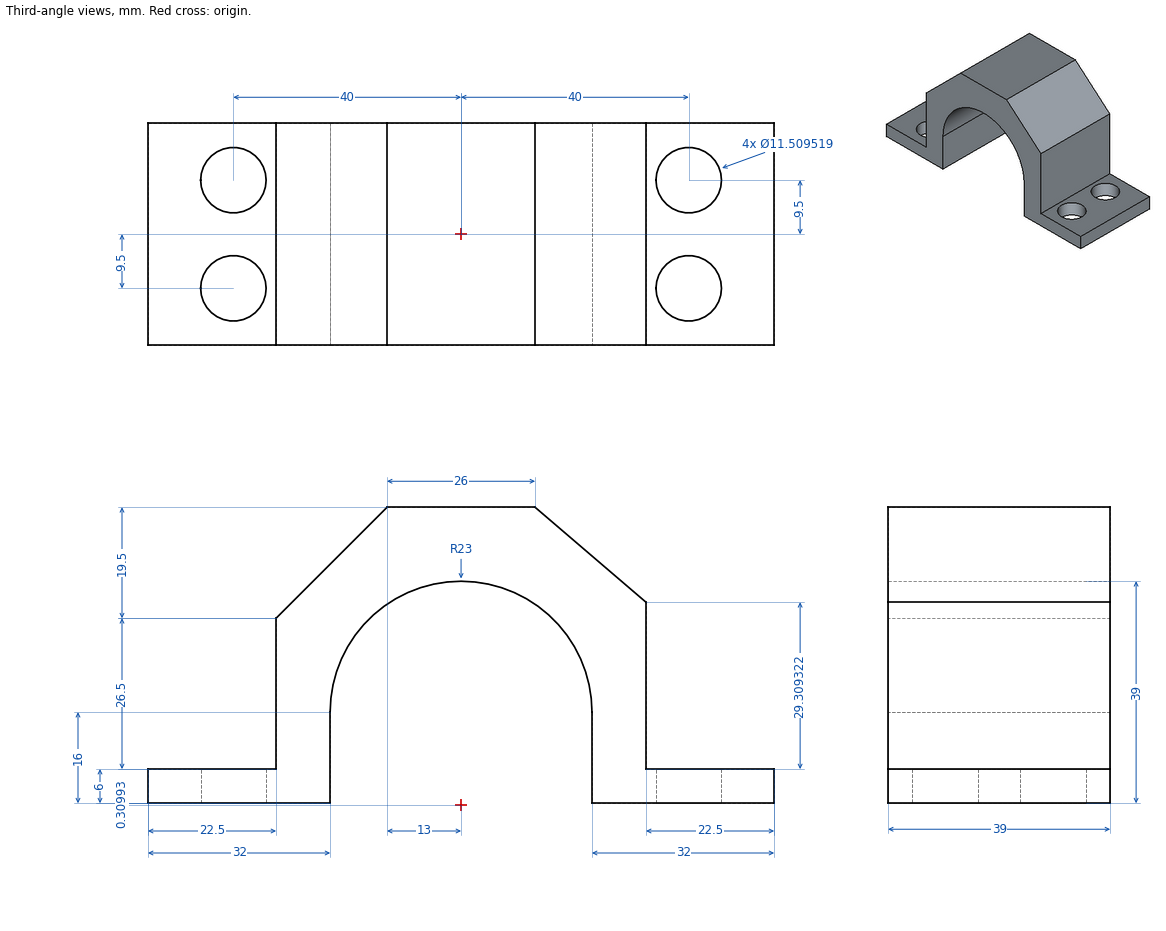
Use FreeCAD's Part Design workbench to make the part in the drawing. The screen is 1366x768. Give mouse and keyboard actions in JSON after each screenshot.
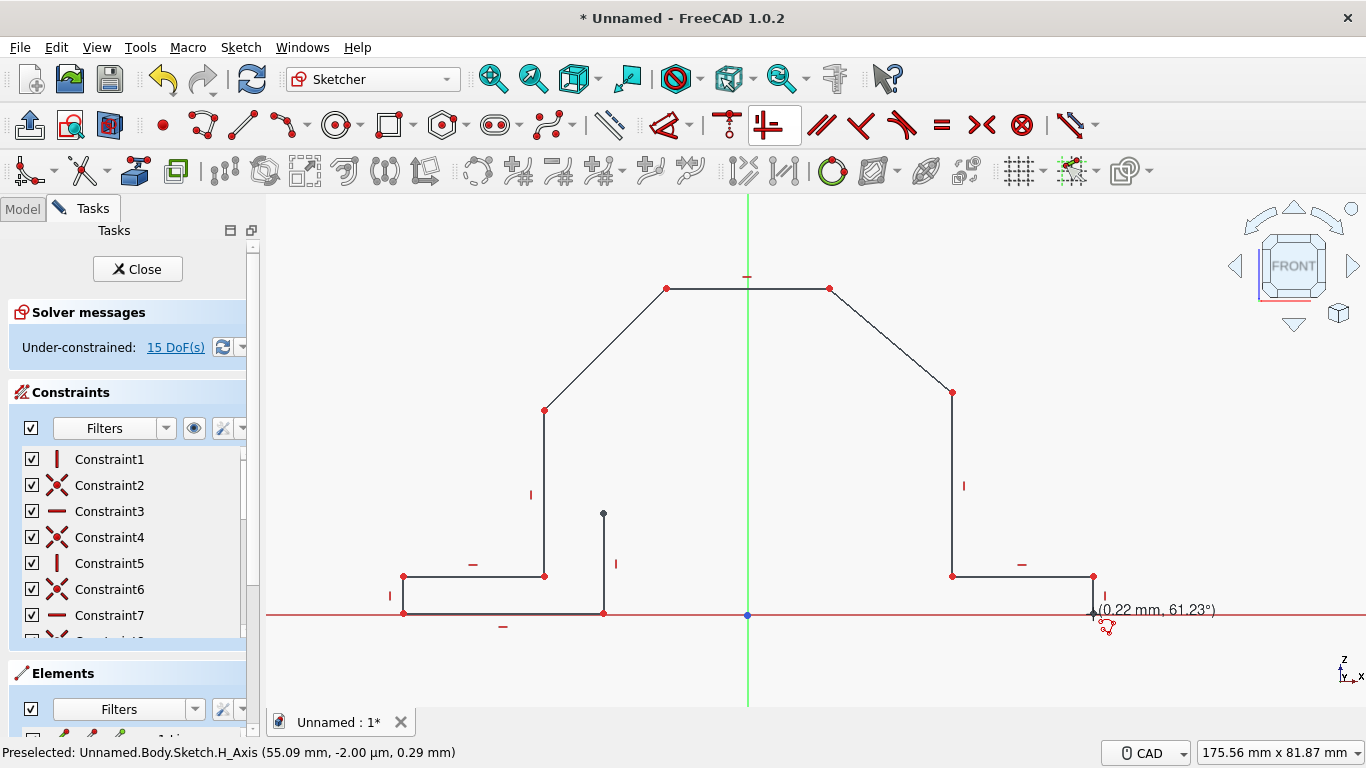
{"action": "scroll", "coordinate": [892, 614], "scroll_direction": "up", "scroll_amount": 11}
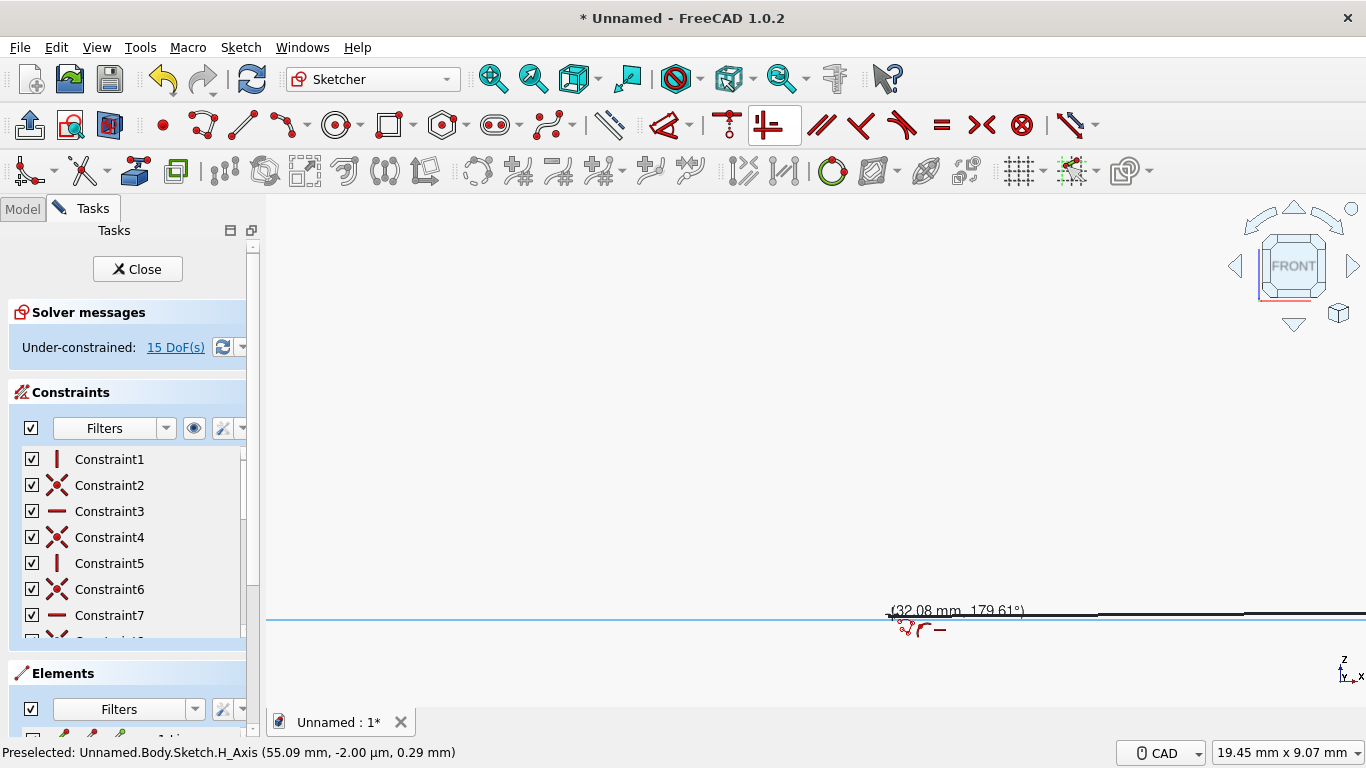
{"action": "left_click", "coordinate": [888, 603]}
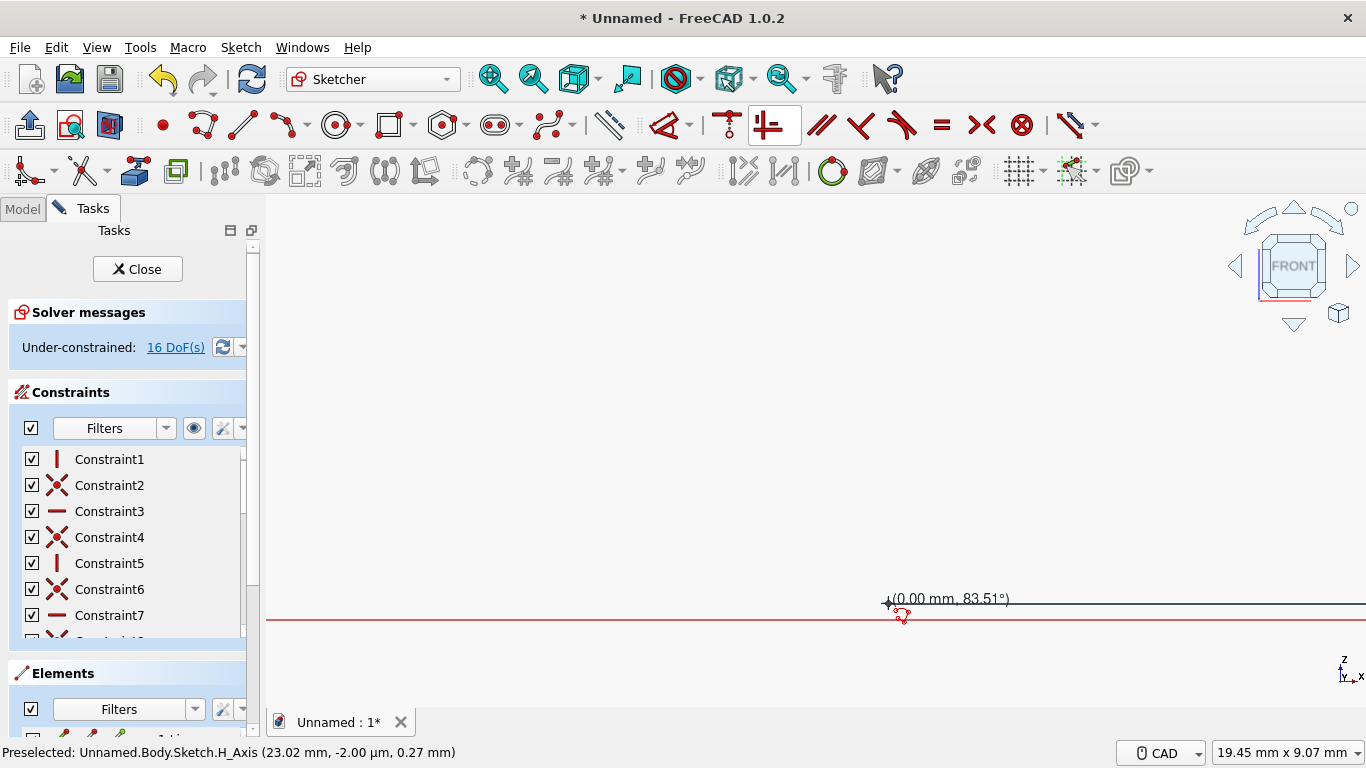
{"action": "scroll", "coordinate": [892, 614], "scroll_direction": "down", "scroll_amount": 11}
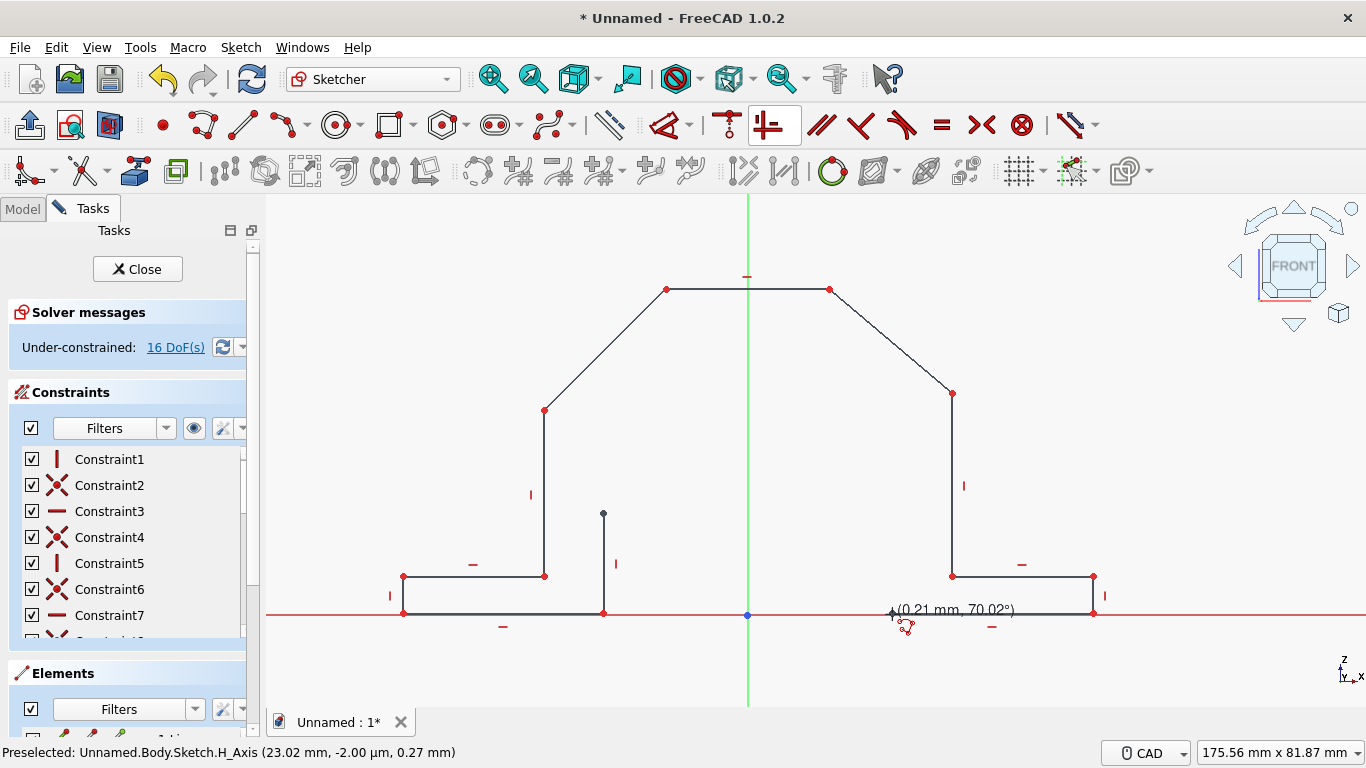
{"action": "left_click", "coordinate": [892, 513]}
{"action": "right_click", "coordinate": [892, 513]}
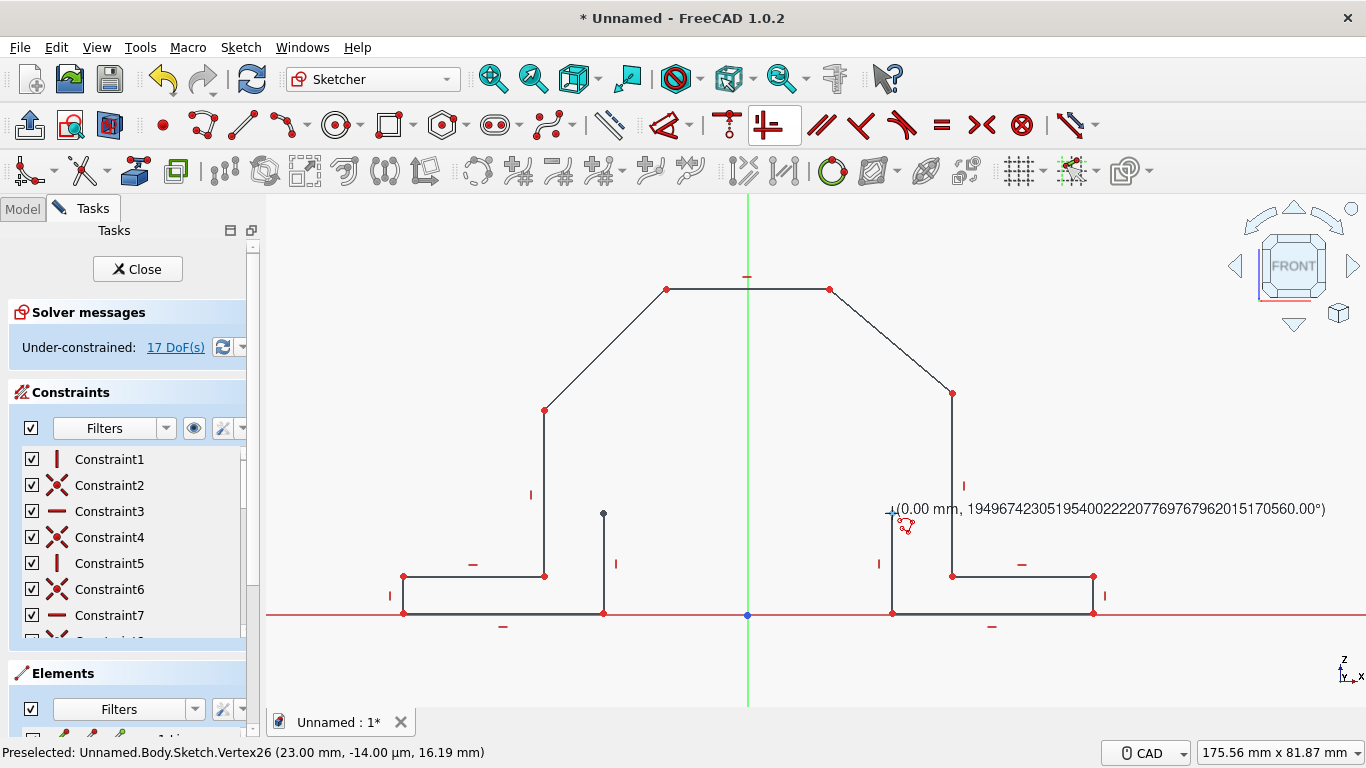
{"action": "left_click", "coordinate": [284, 126]}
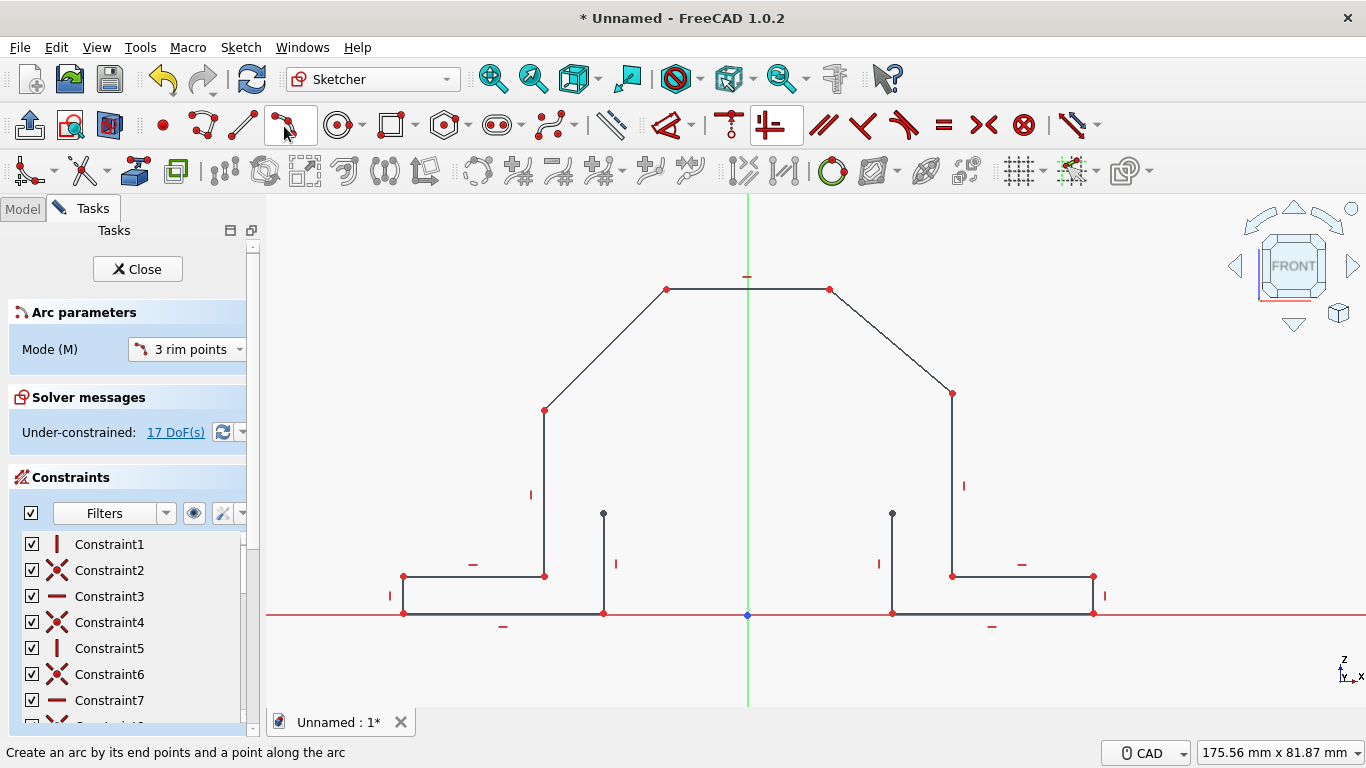
{"action": "left_click", "coordinate": [892, 514]}
{"action": "left_click", "coordinate": [604, 514]}
{"action": "left_click", "coordinate": [792, 376]}
{"action": "key", "text": "Escape"}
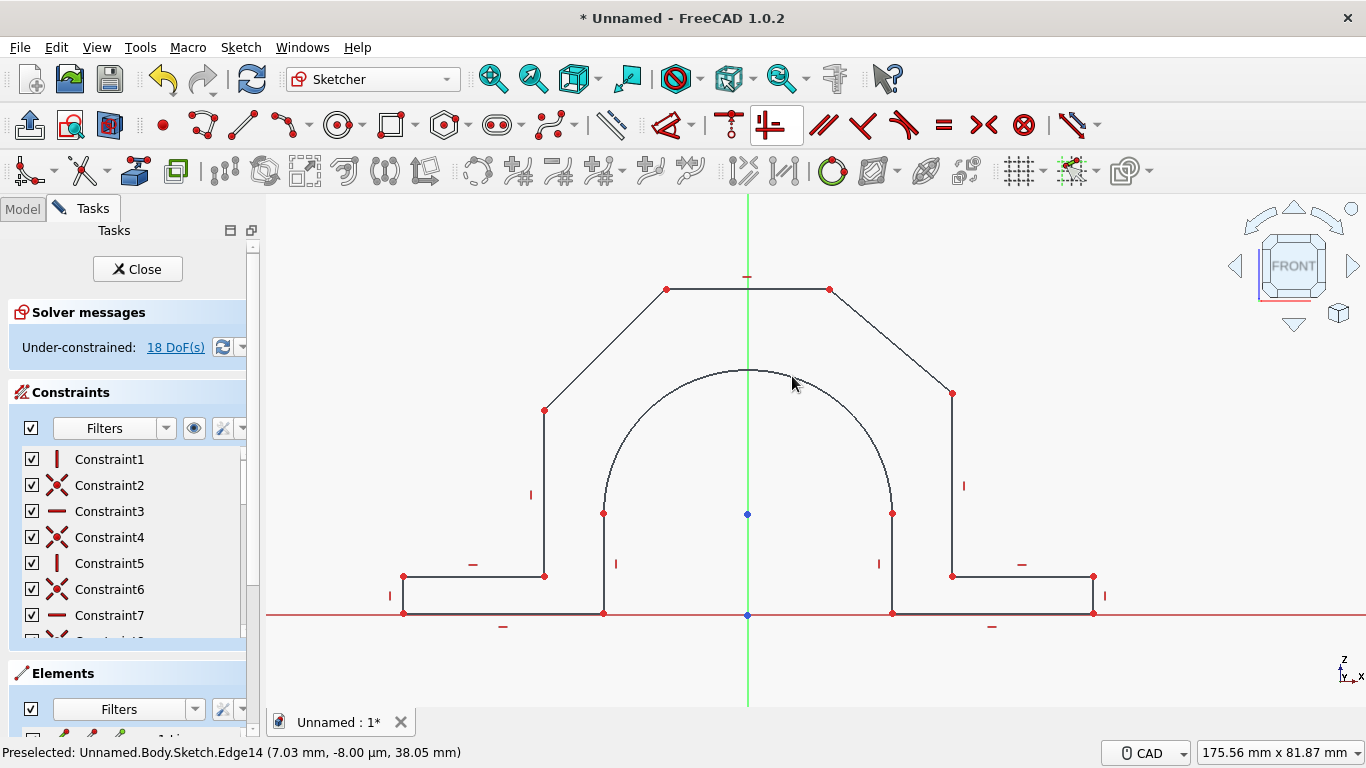
{"action": "left_click", "coordinate": [604, 544]}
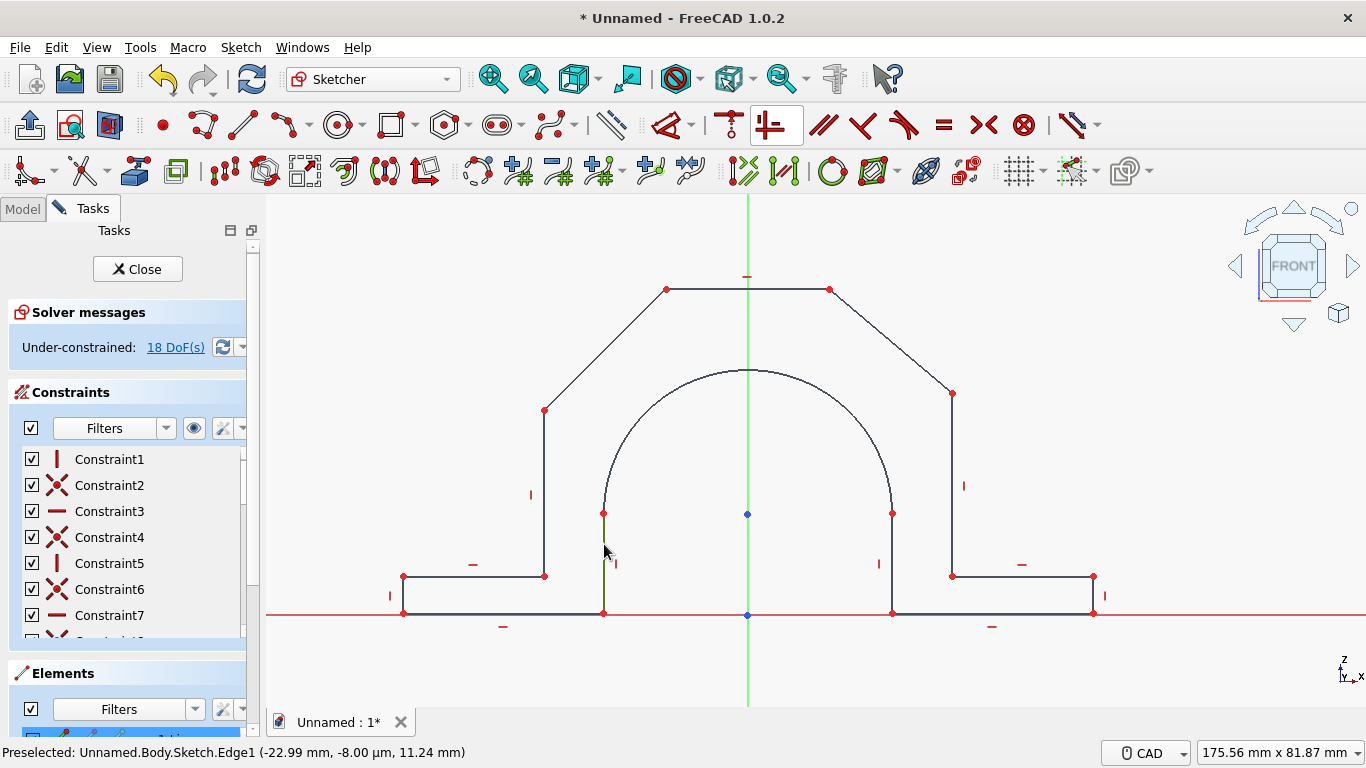
{"action": "left_click", "coordinate": [833, 398]}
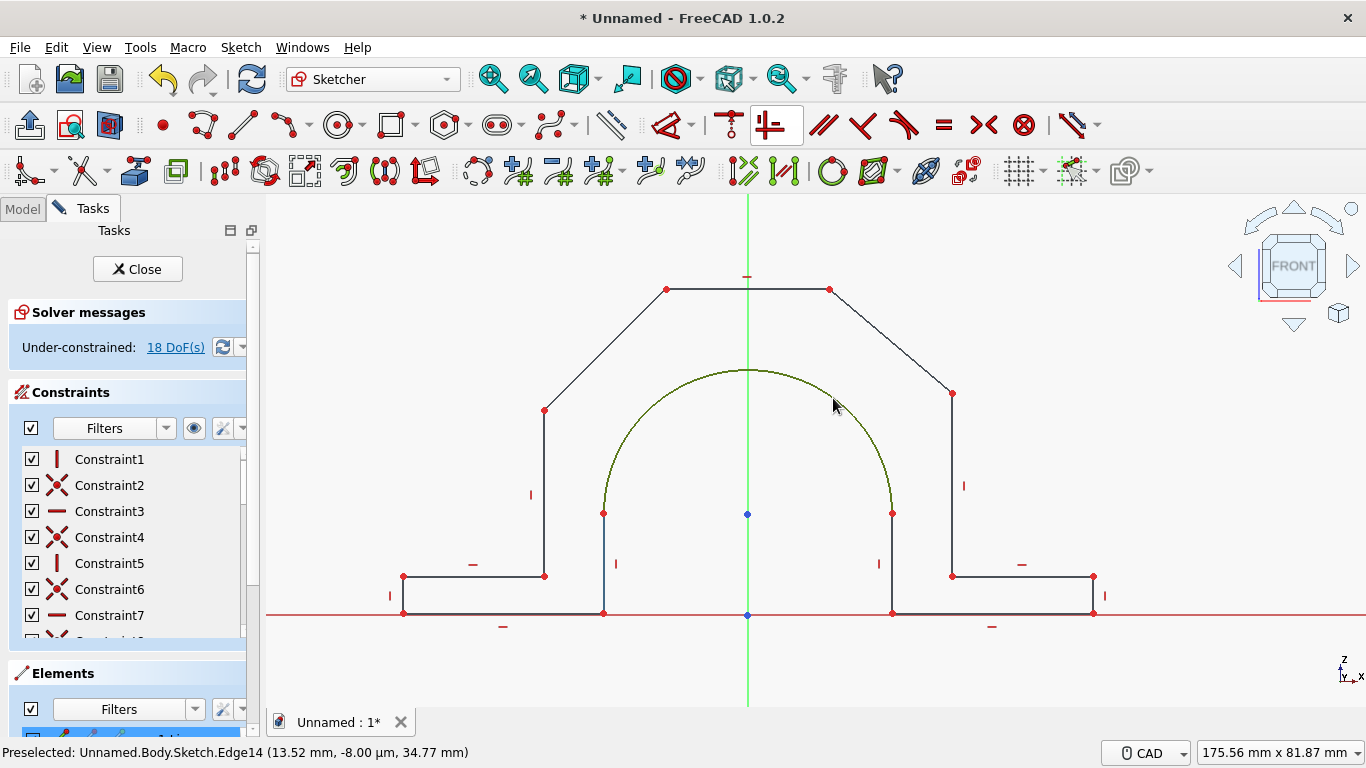
{"action": "left_click", "coordinate": [904, 126]}